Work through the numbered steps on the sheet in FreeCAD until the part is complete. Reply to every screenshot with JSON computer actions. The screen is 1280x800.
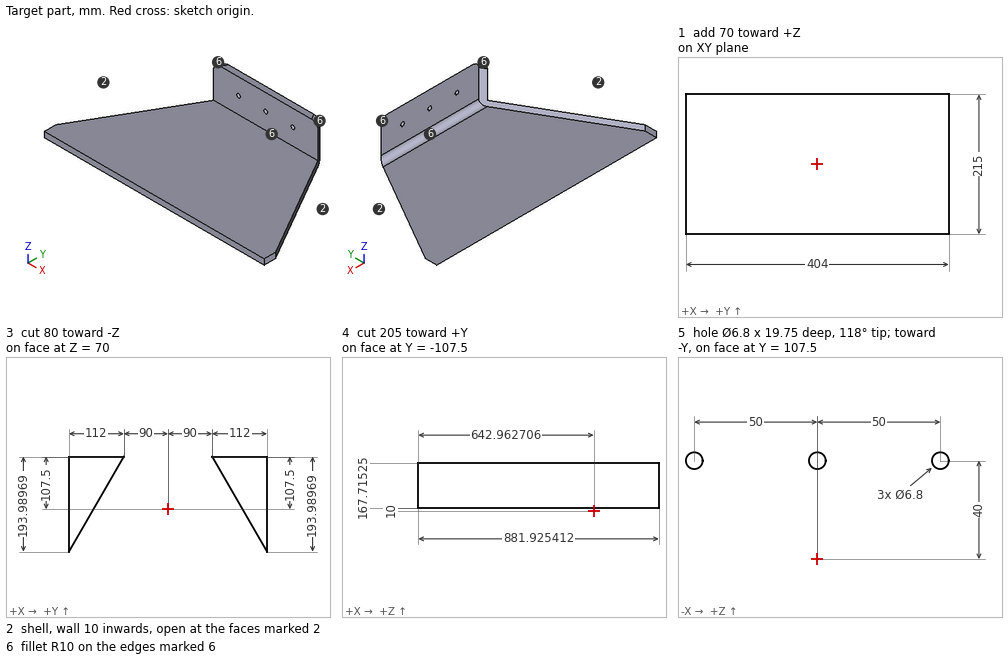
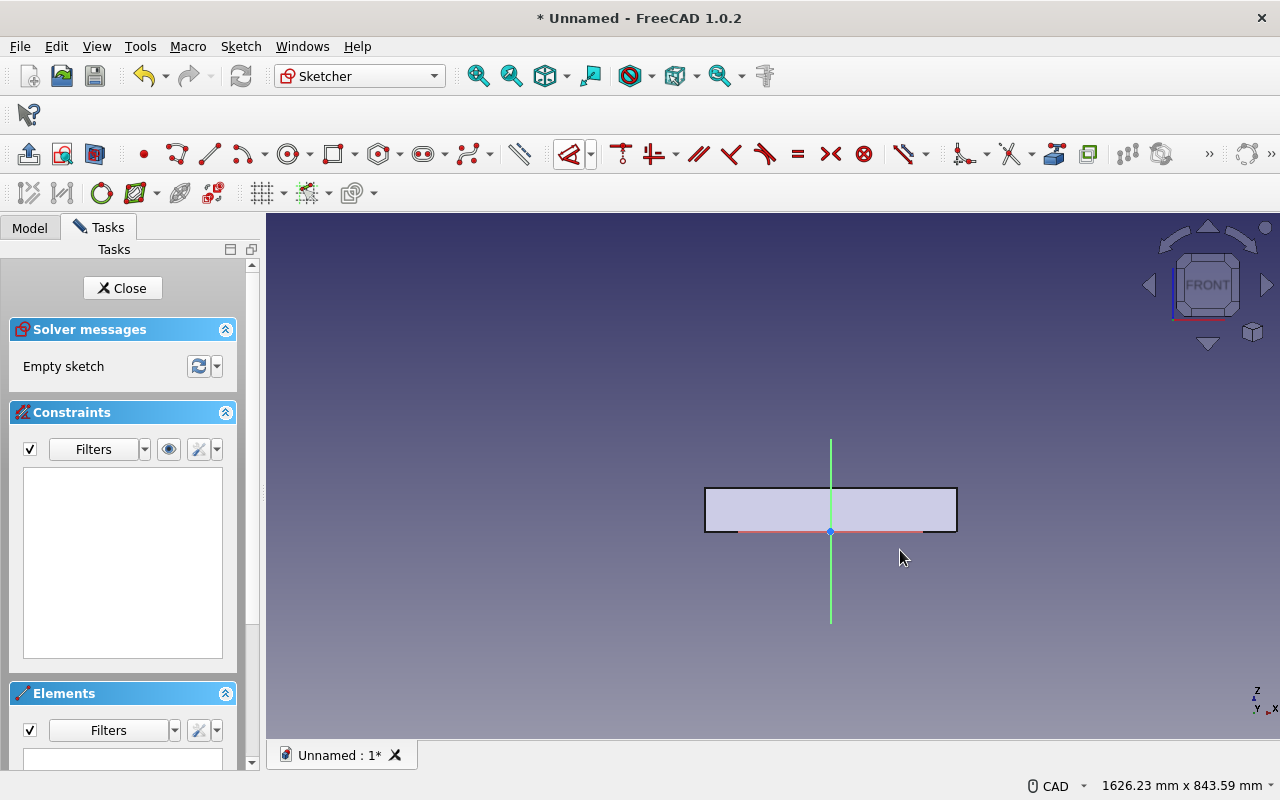
{"action": "left_click", "coordinate": [332, 154]}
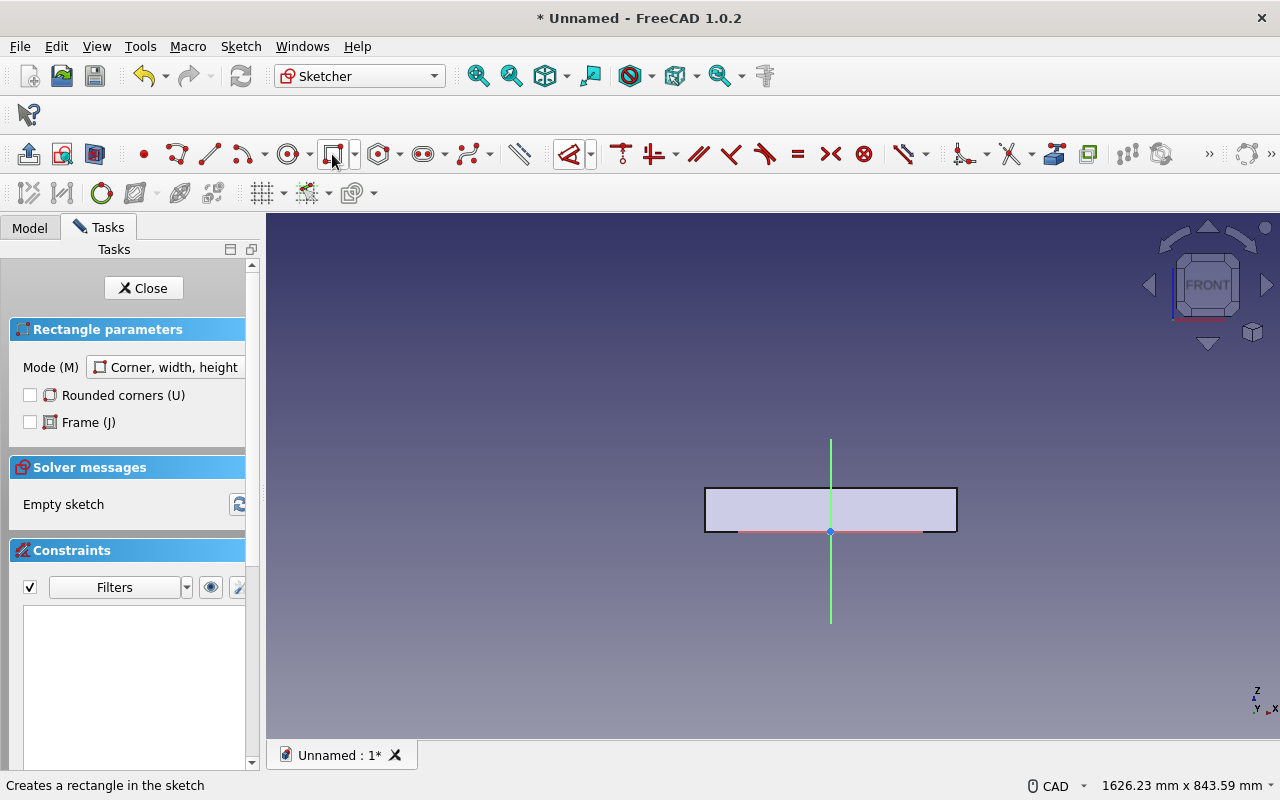
{"action": "left_click", "coordinate": [430, 421]}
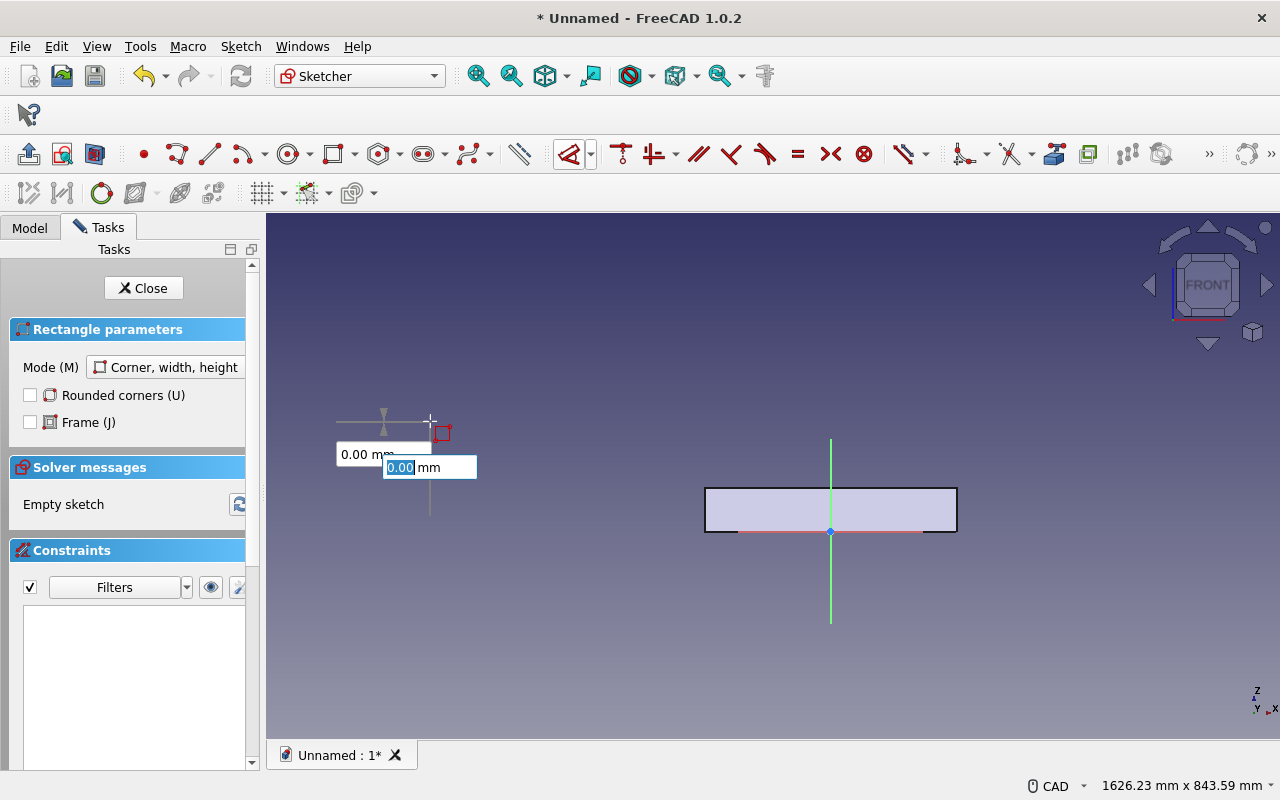
{"action": "scroll", "coordinate": [980, 525], "scroll_direction": "up", "scroll_amount": 5}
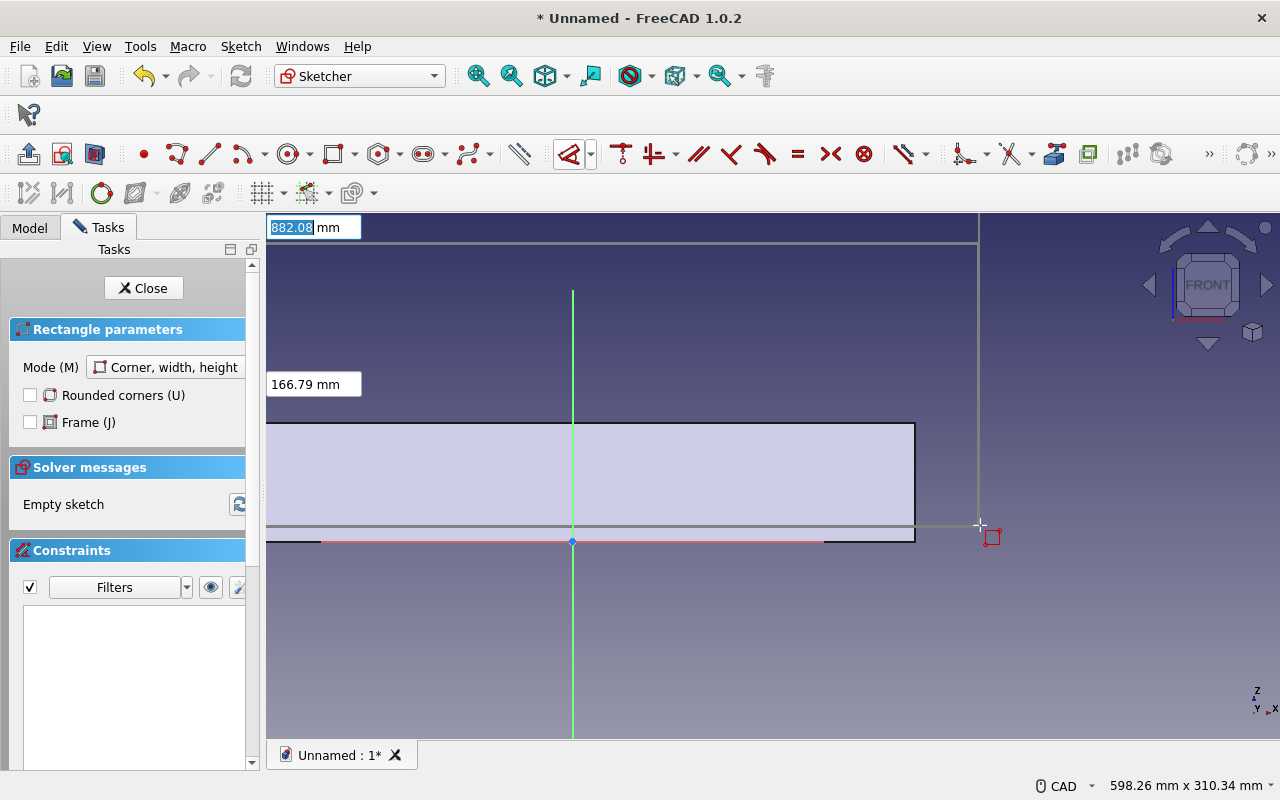
{"action": "left_click", "coordinate": [978, 525]}
{"action": "key", "text": "Escape"}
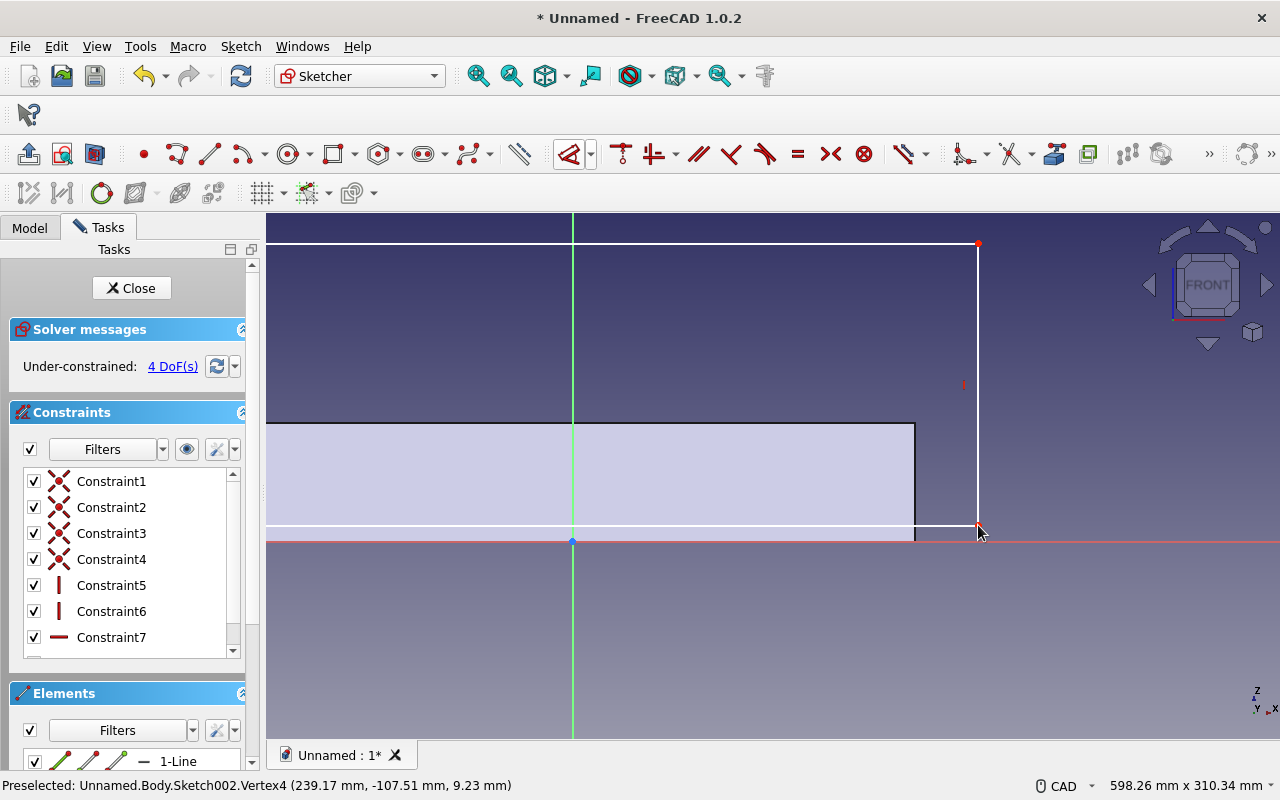
{"action": "scroll", "coordinate": [980, 525], "scroll_direction": "down", "scroll_amount": 5}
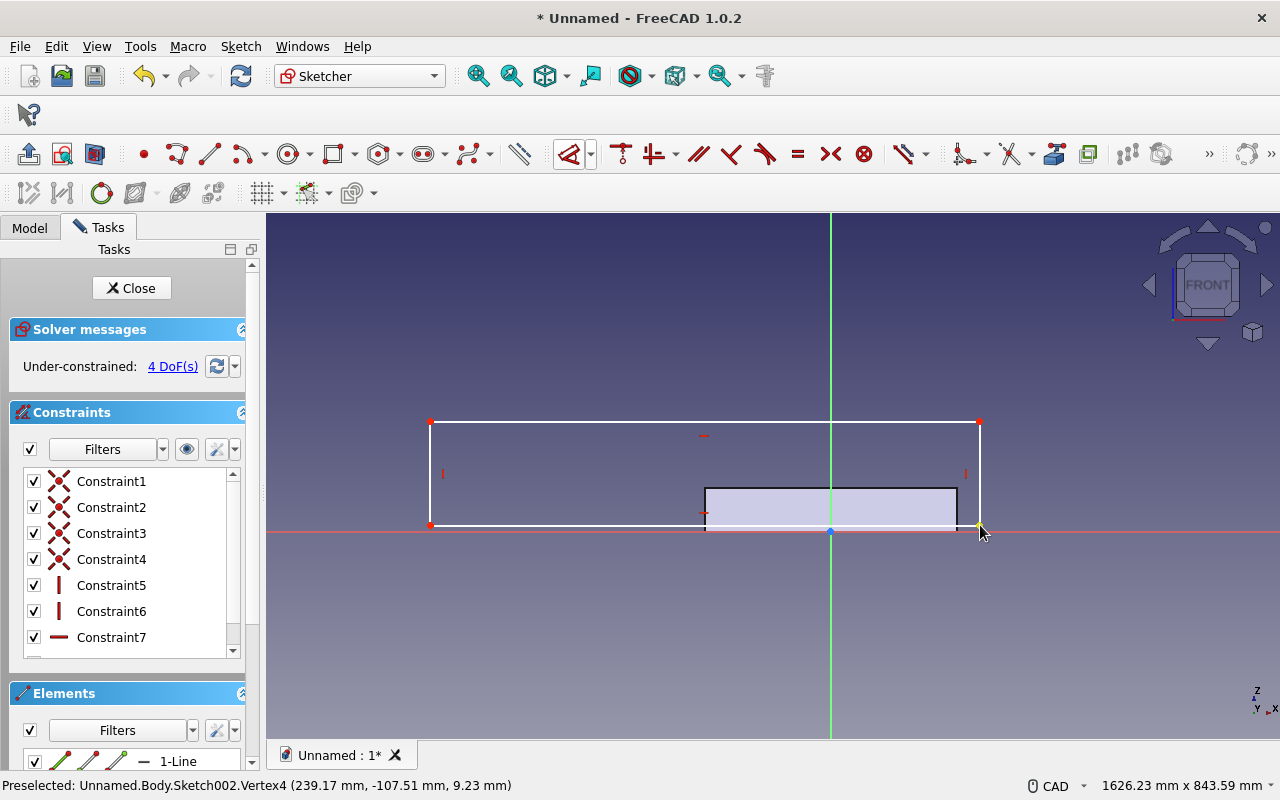
{"action": "scroll", "coordinate": [430, 526], "scroll_direction": "up", "scroll_amount": 10}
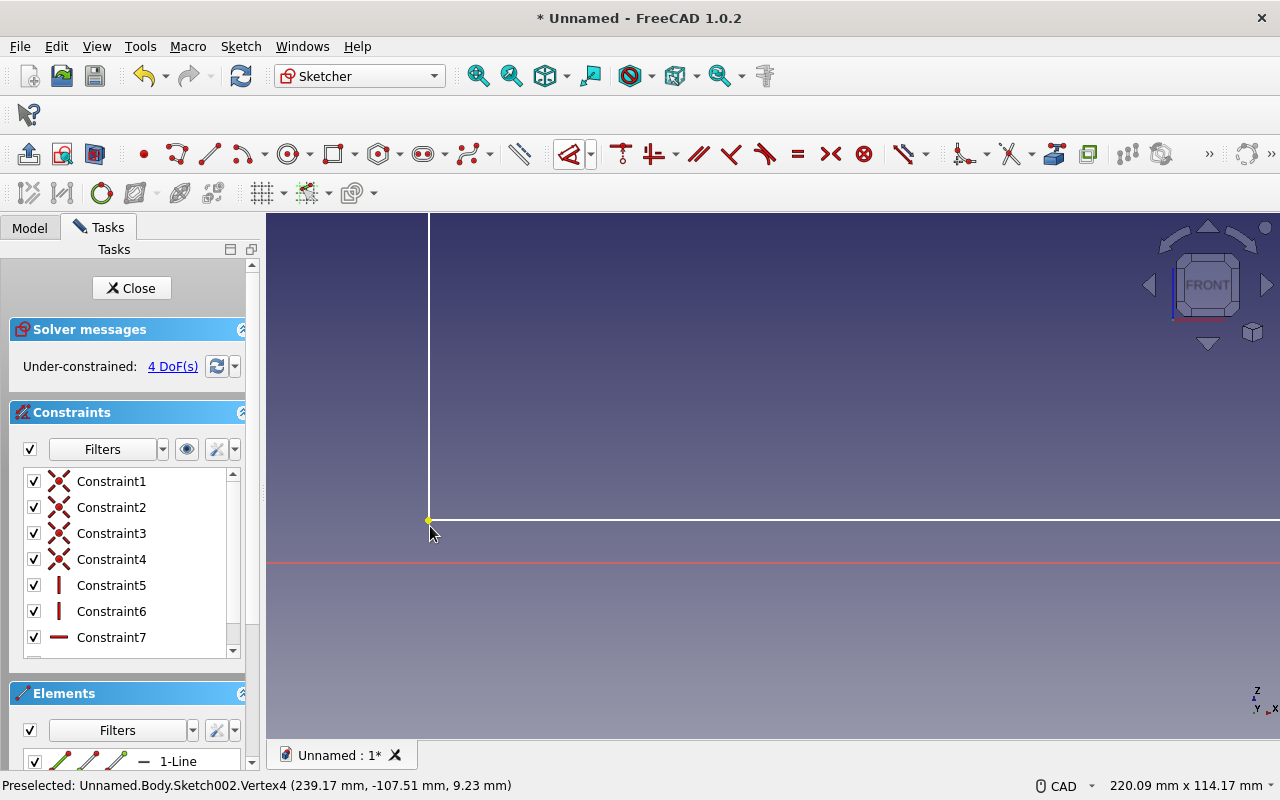
{"action": "left_click", "coordinate": [429, 520]}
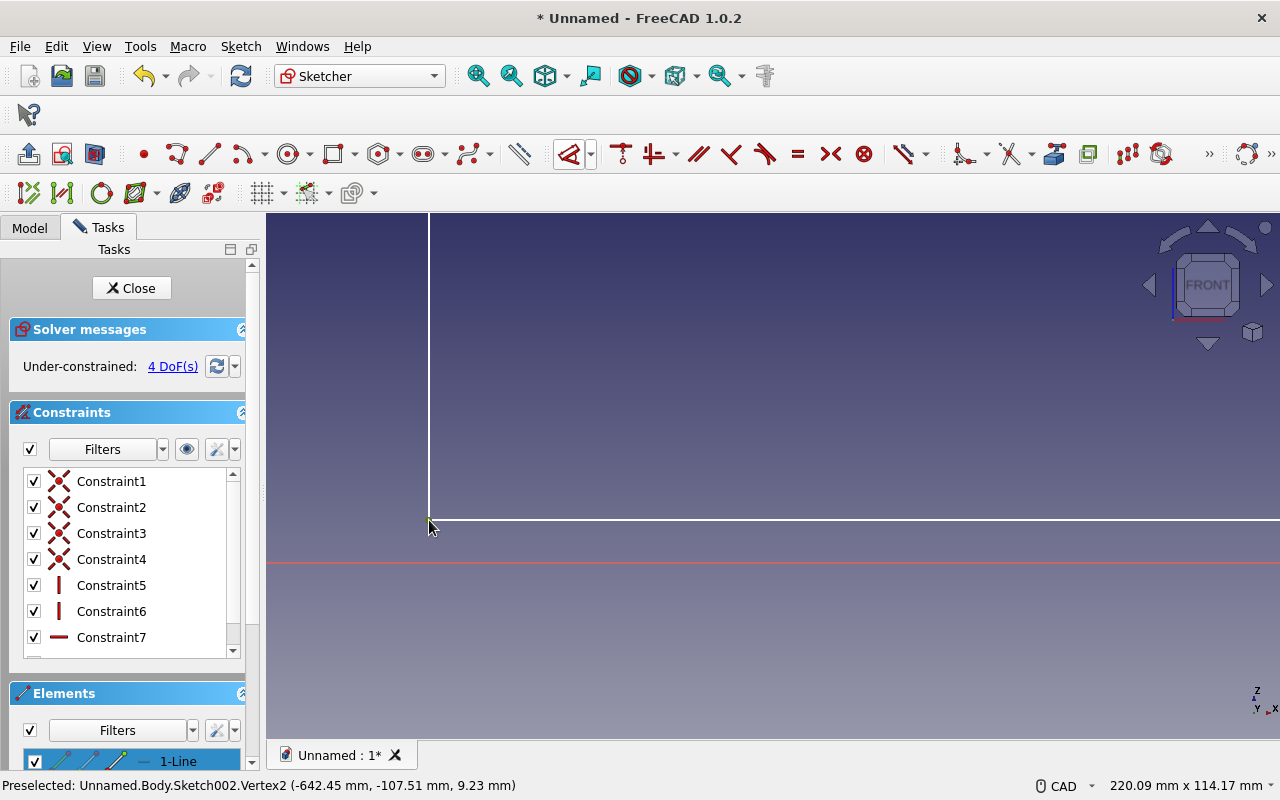
{"action": "left_click", "coordinate": [590, 154]}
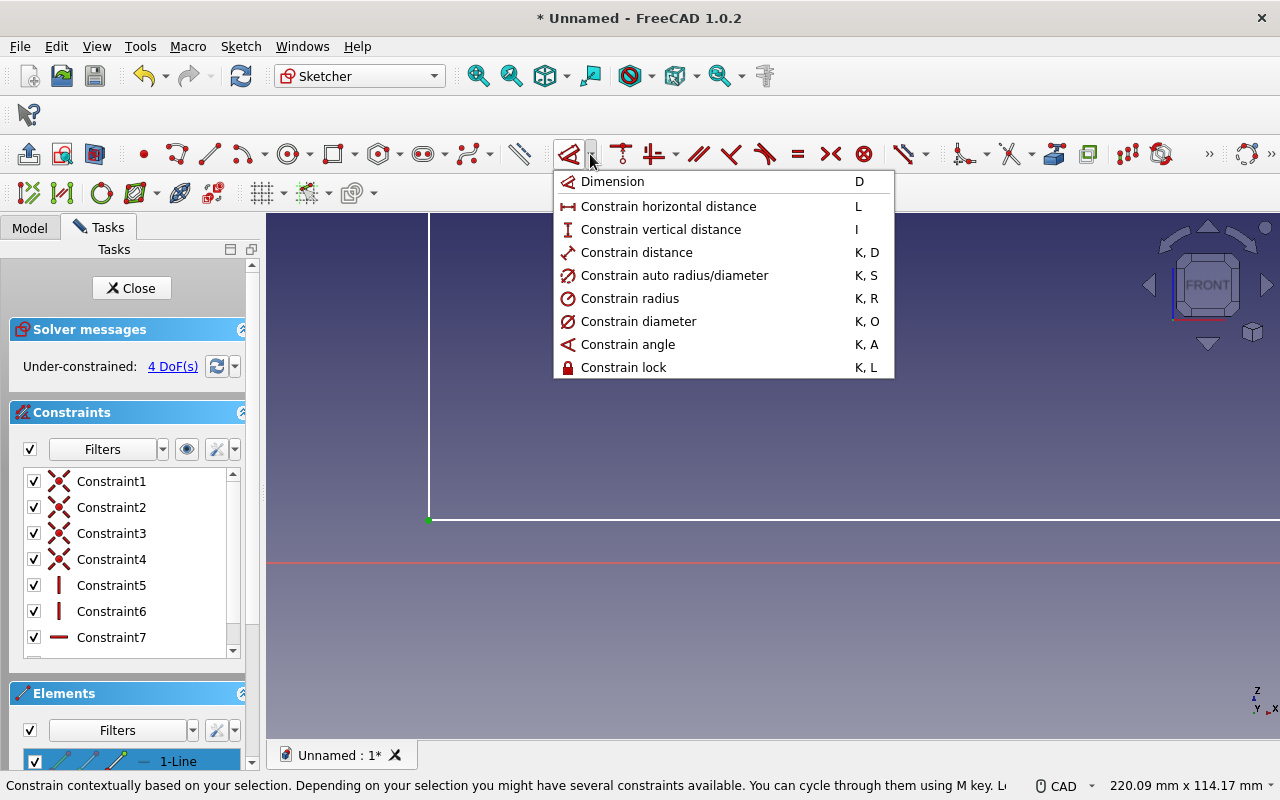
{"action": "left_click", "coordinate": [724, 230]}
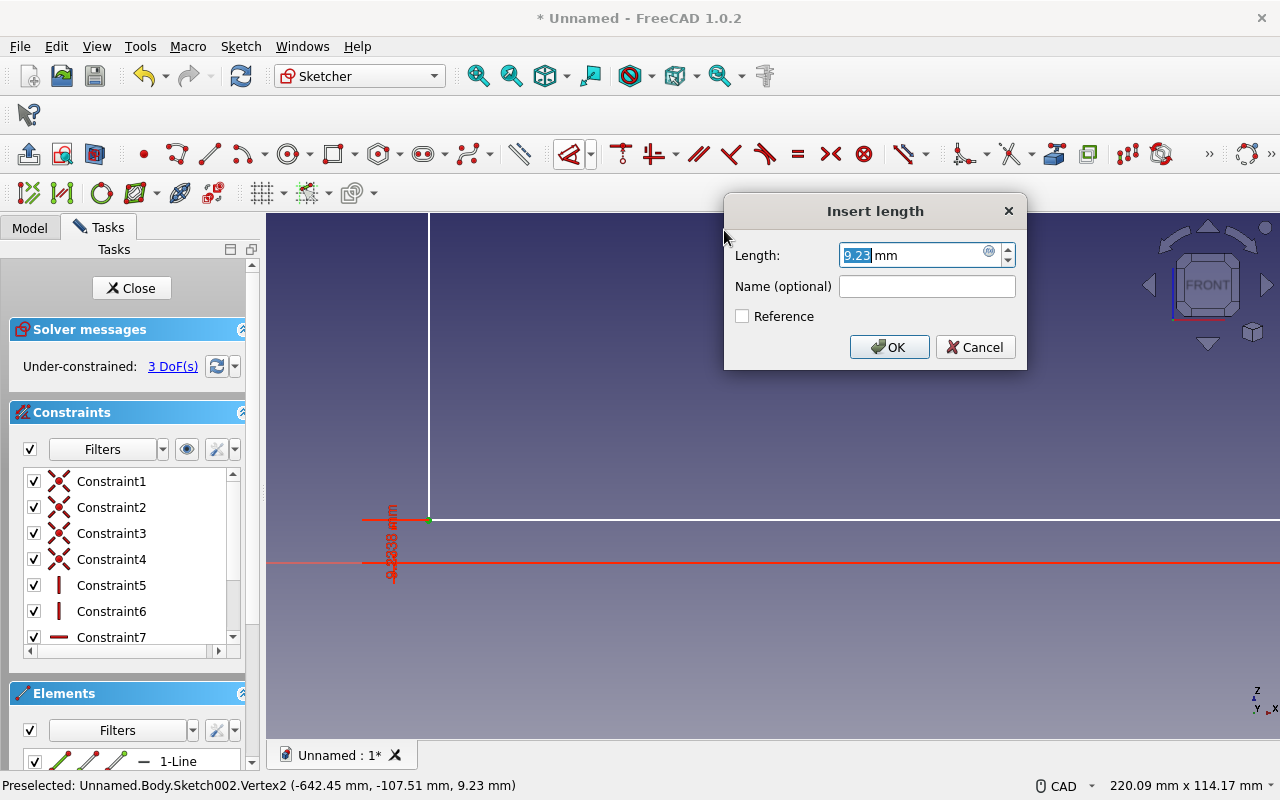
{"action": "type", "text": "10"}
{"action": "key", "text": "Return"}